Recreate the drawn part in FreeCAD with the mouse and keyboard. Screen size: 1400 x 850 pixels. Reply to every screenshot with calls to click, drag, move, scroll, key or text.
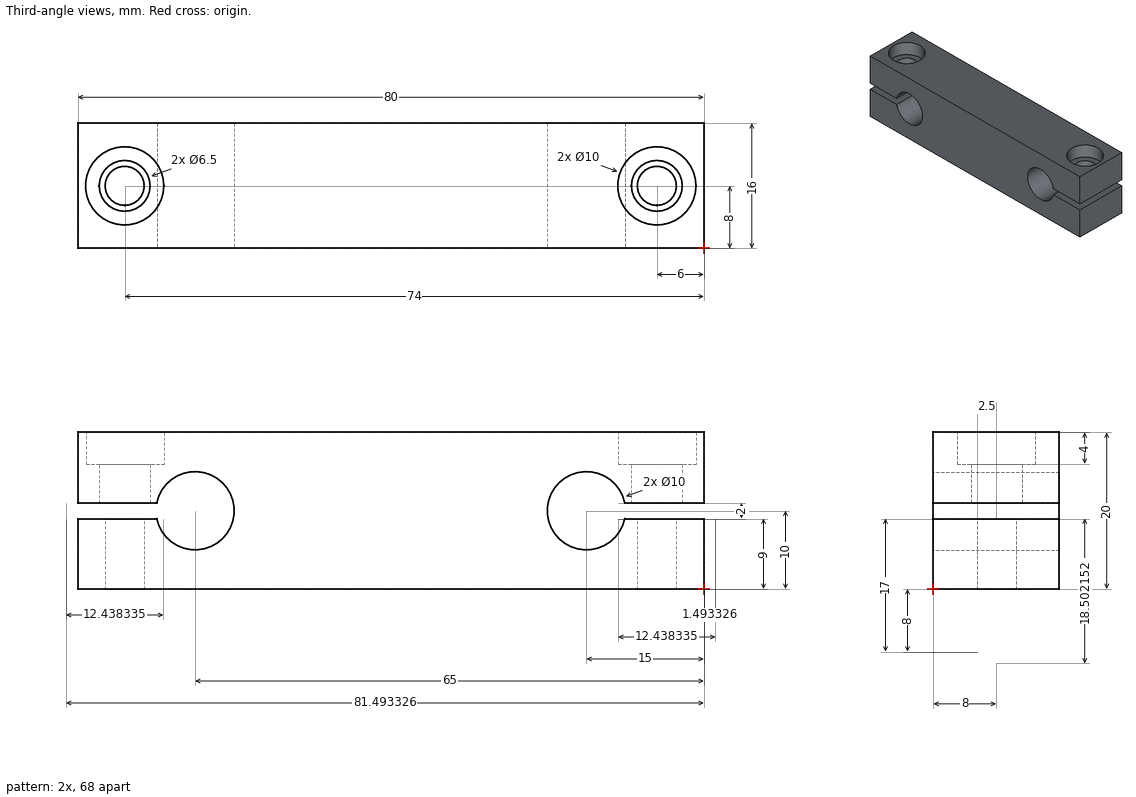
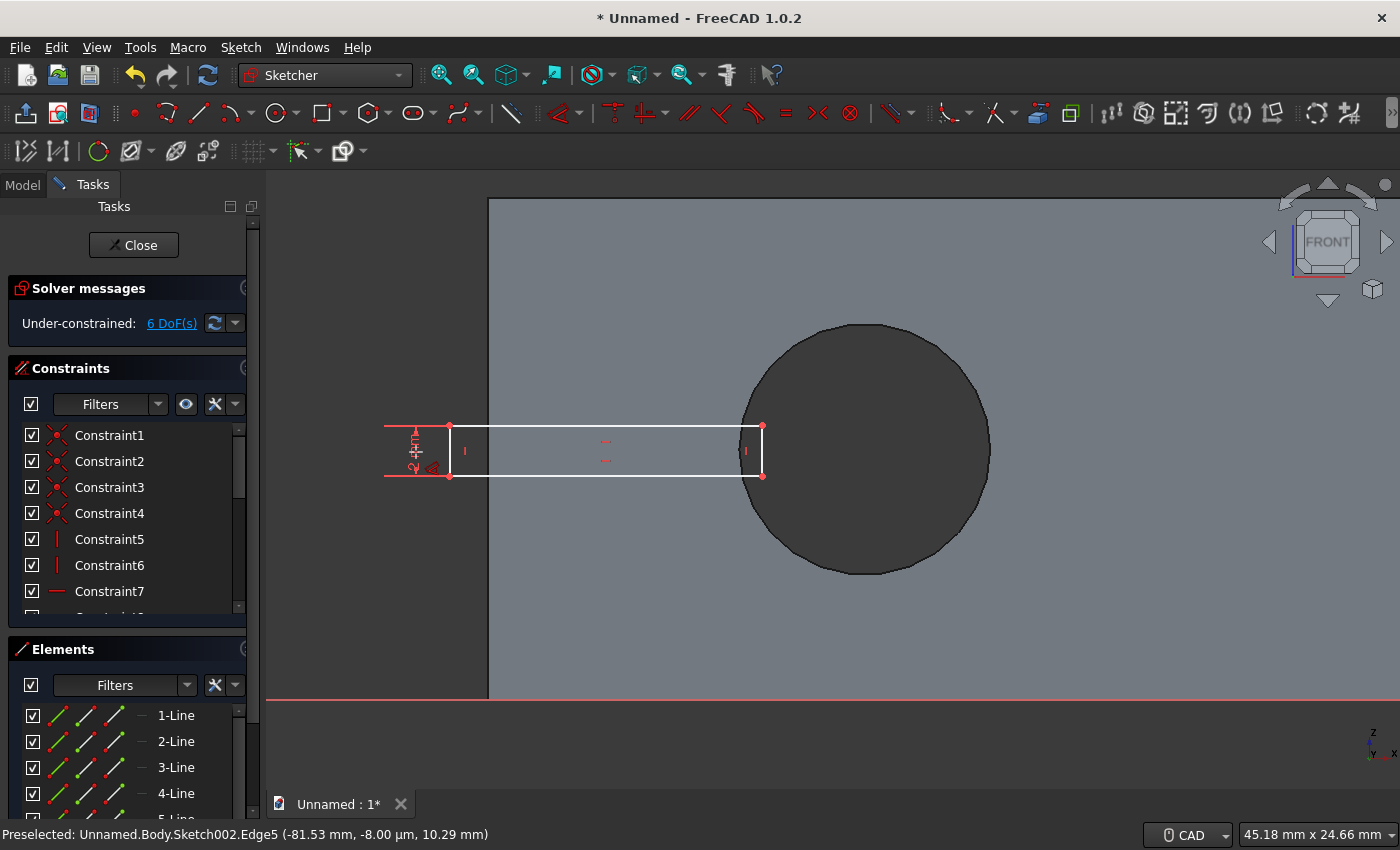
scroll(451, 444, down, 6)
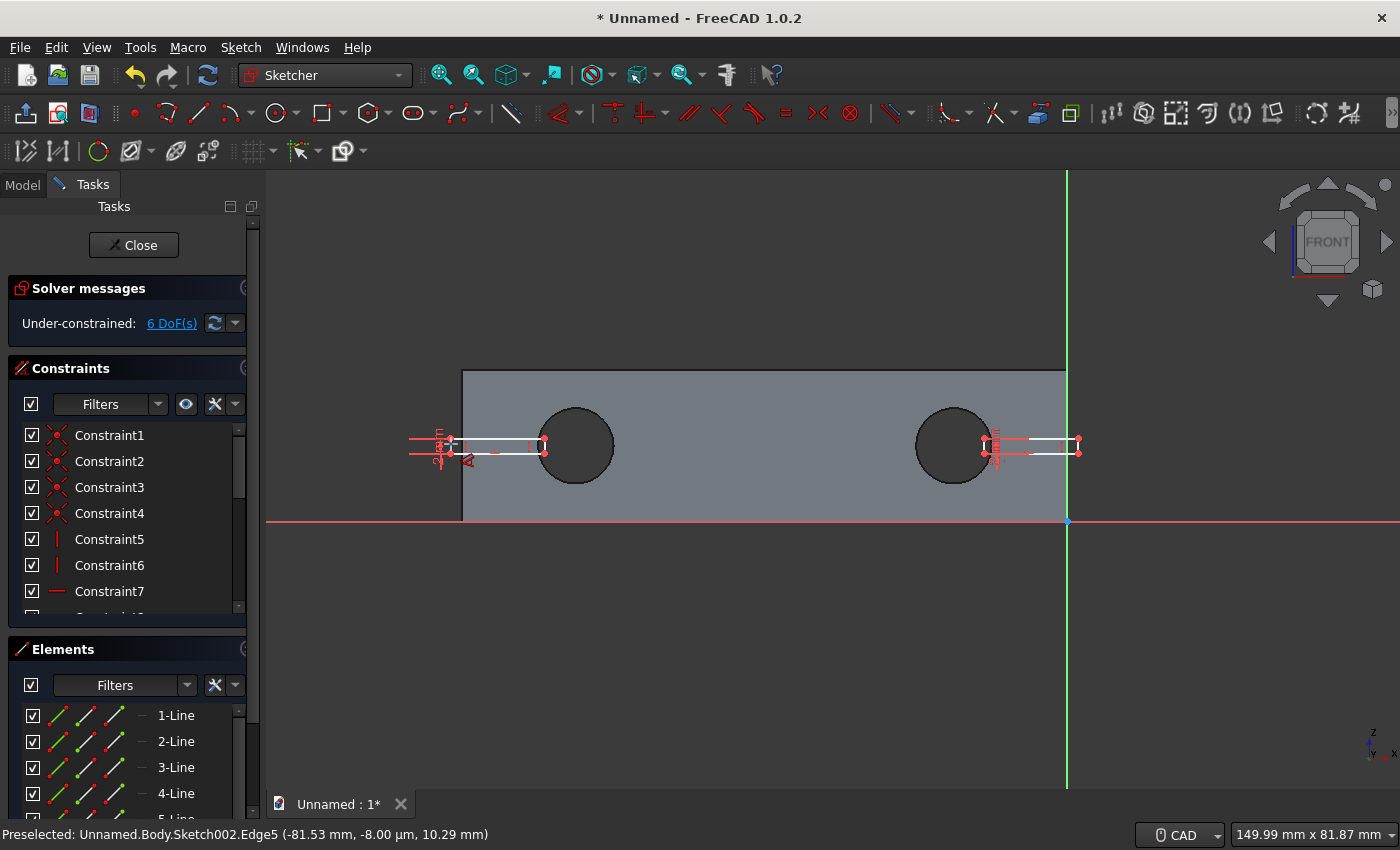
click(984, 454)
click(1101, 488)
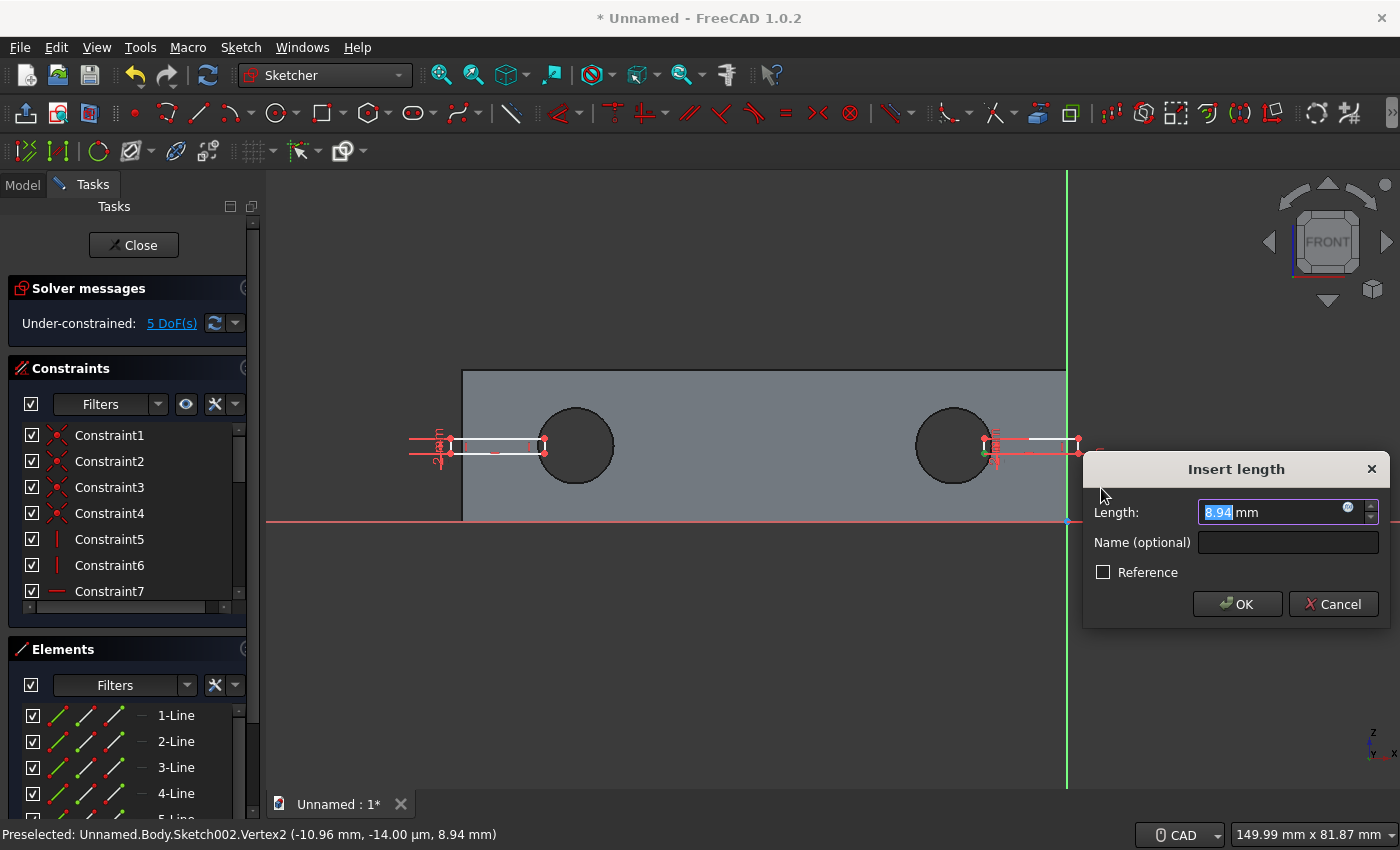
text(9)
key(Return)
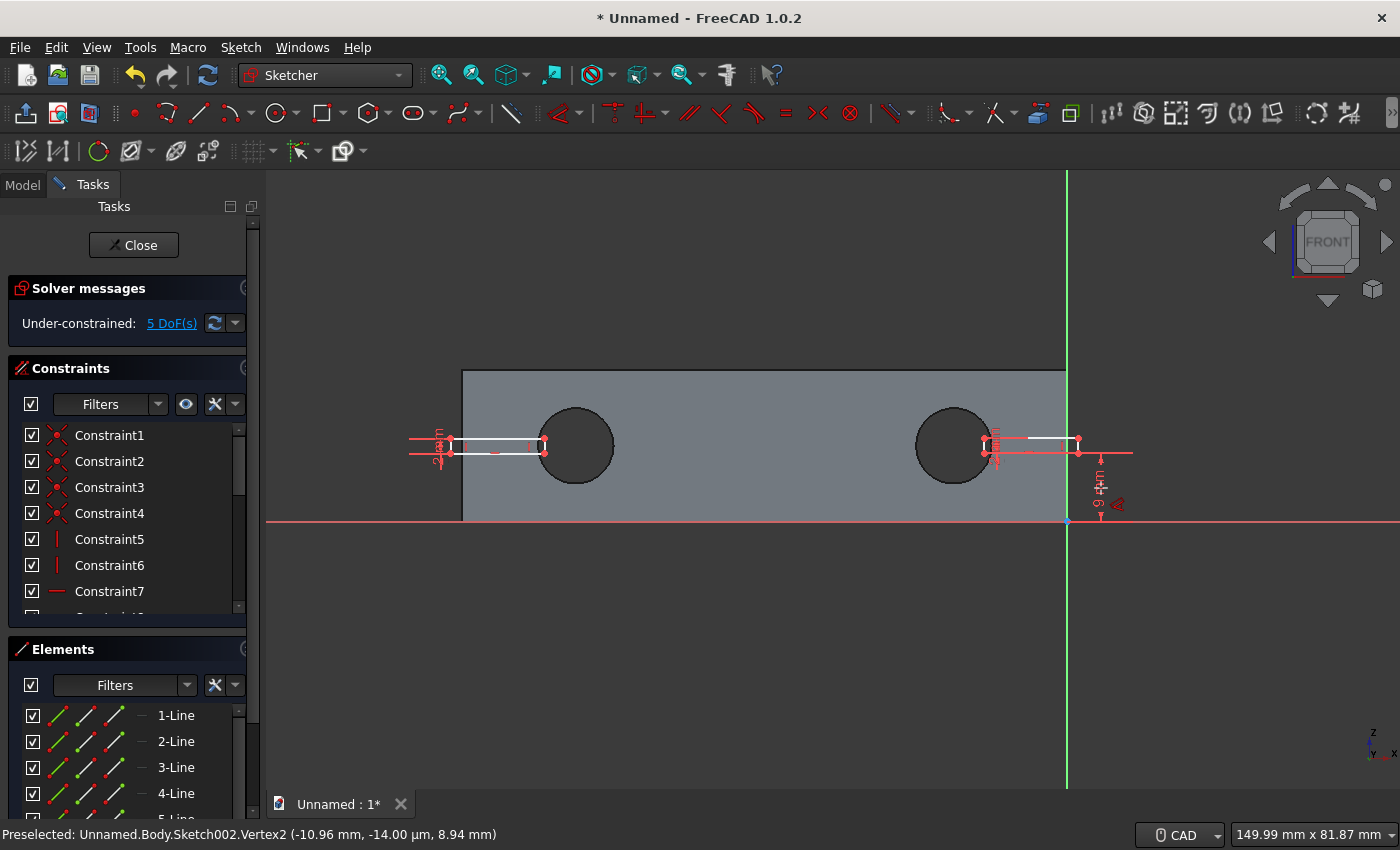
click(451, 454)
click(417, 488)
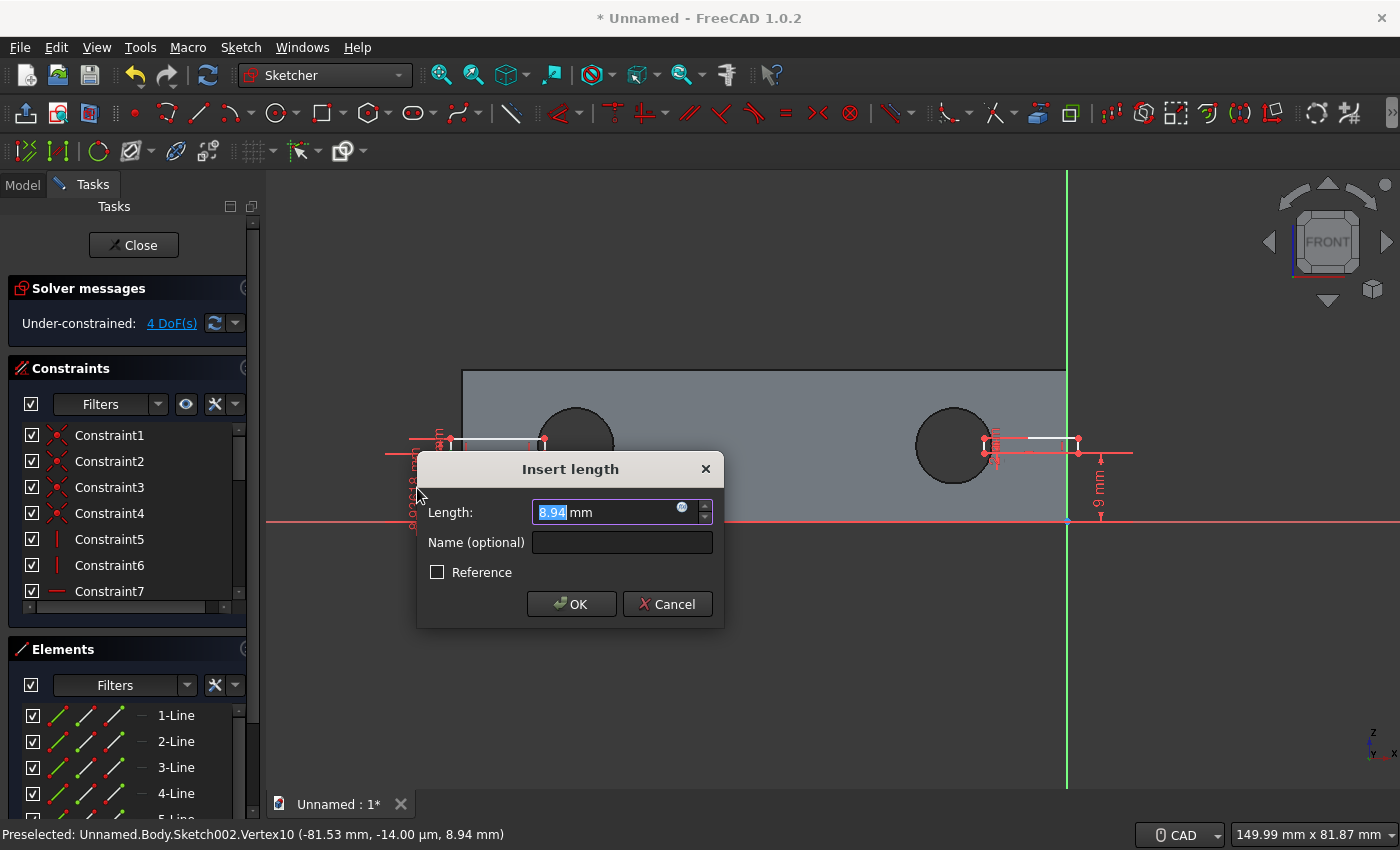
text(9)
key(Return)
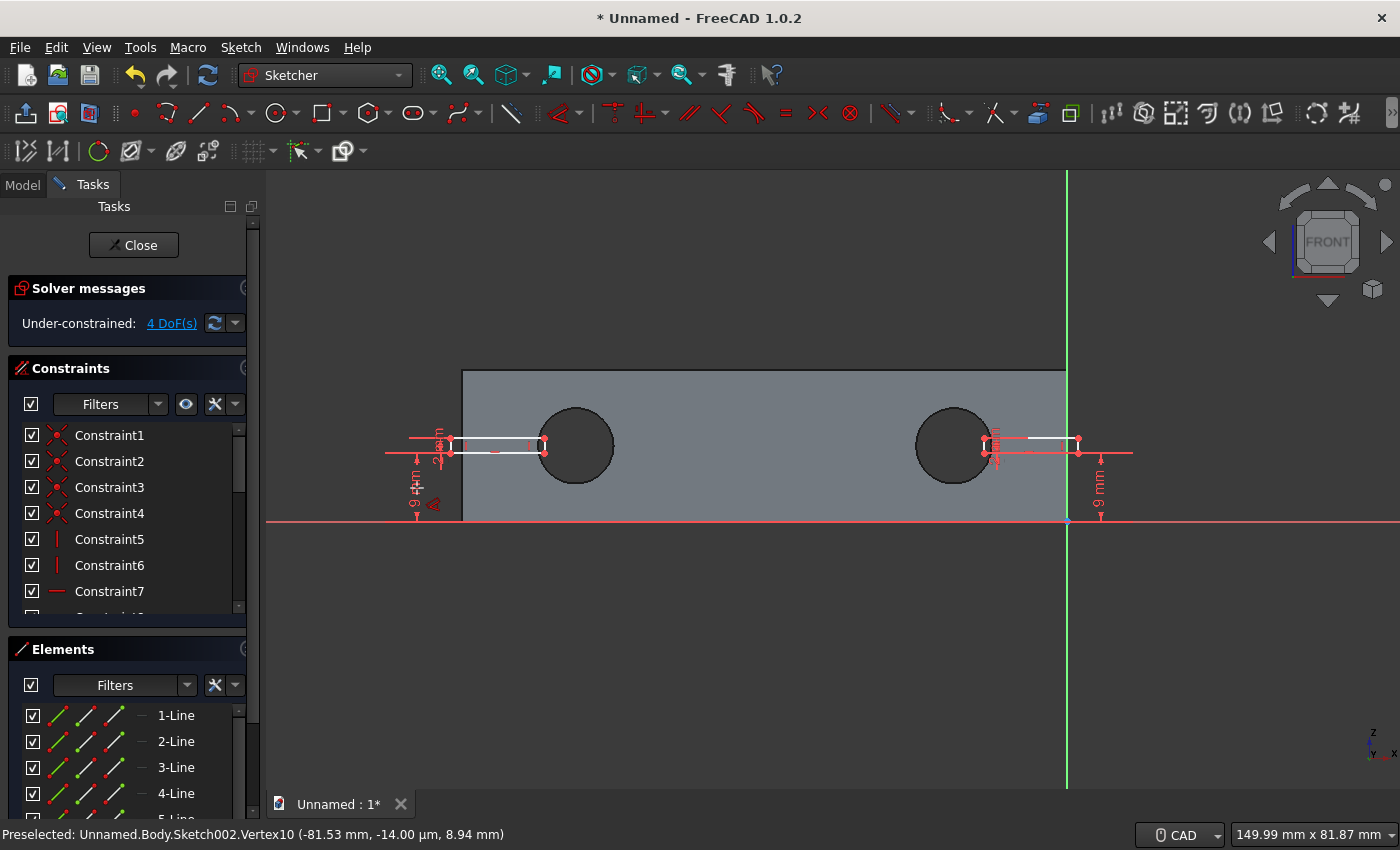
click(1013, 453)
click(1031, 419)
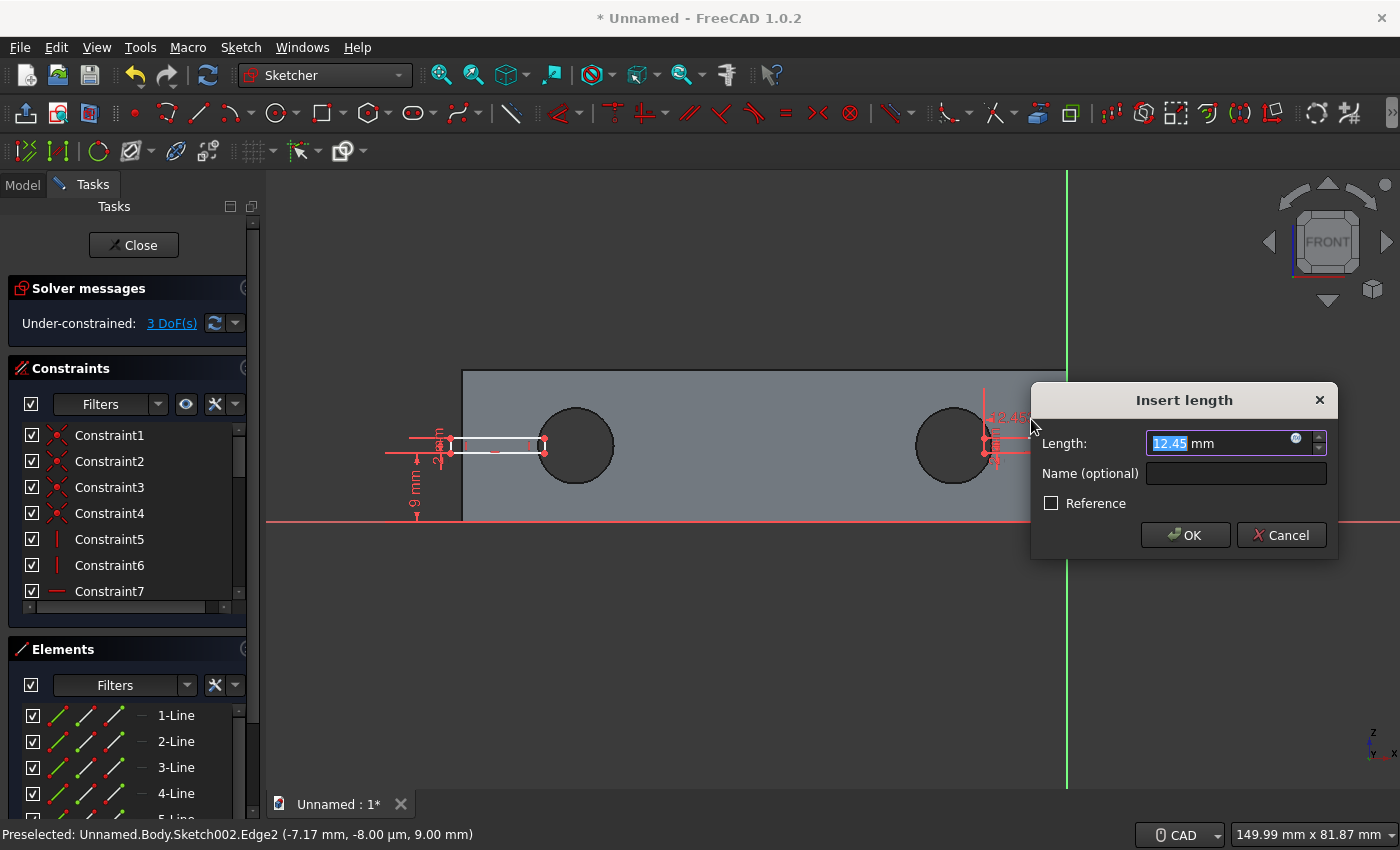
text(12.438335)
key(Return)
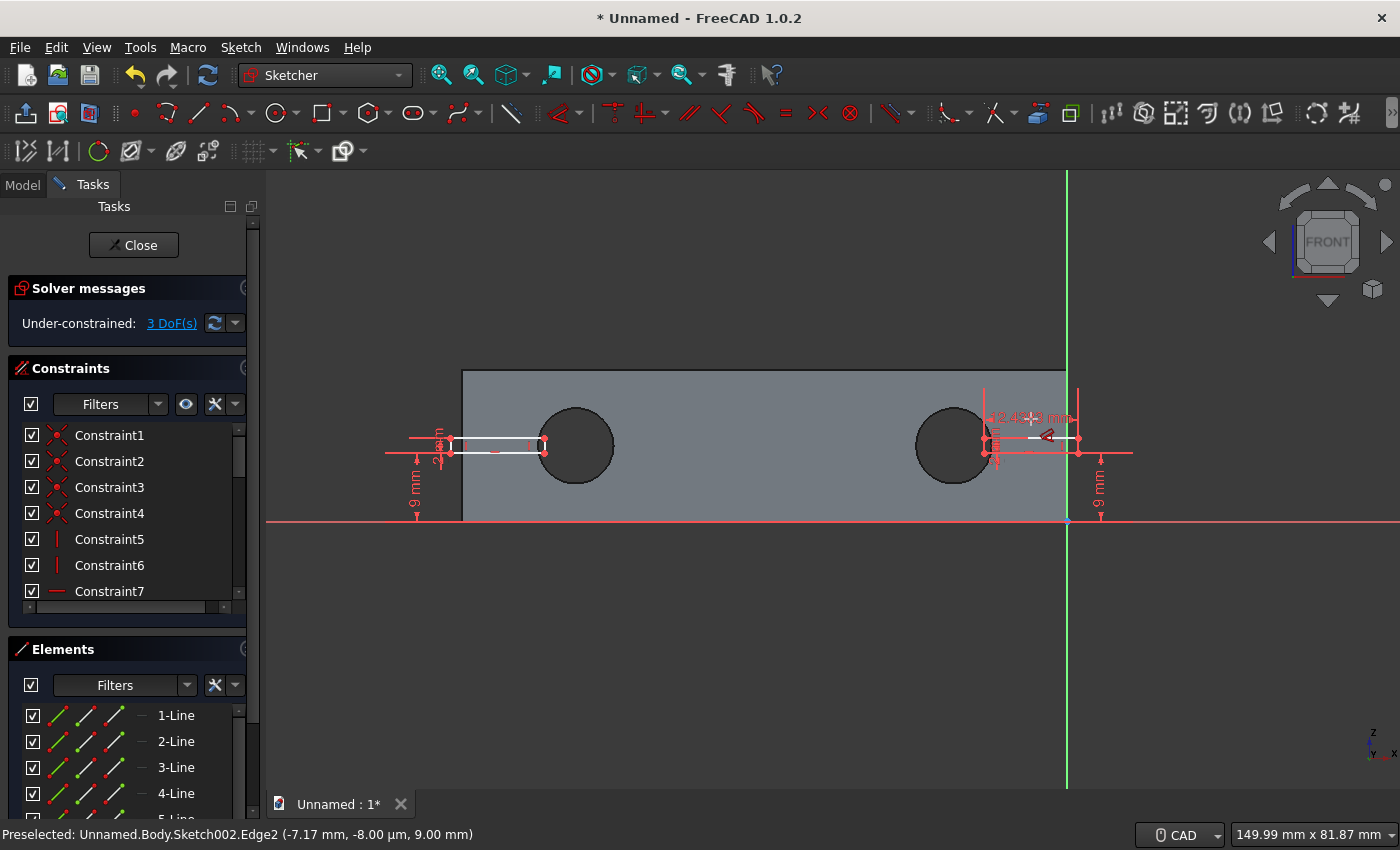
click(479, 453)
click(498, 419)